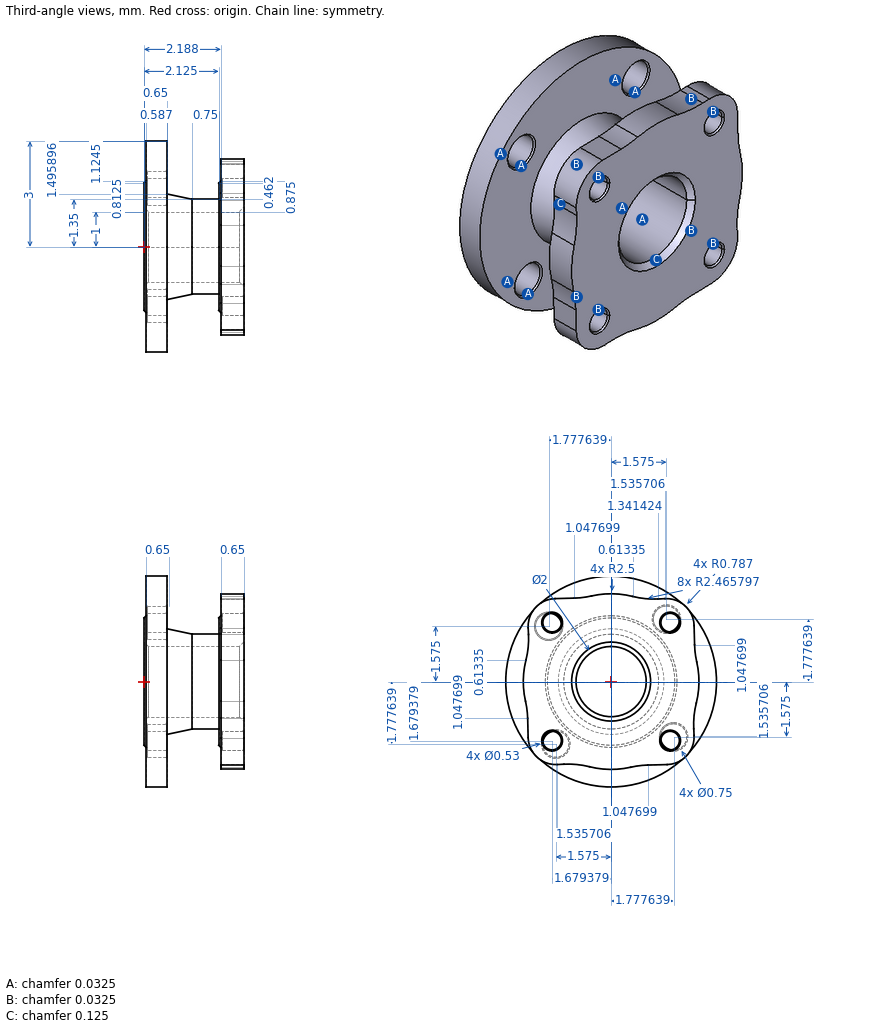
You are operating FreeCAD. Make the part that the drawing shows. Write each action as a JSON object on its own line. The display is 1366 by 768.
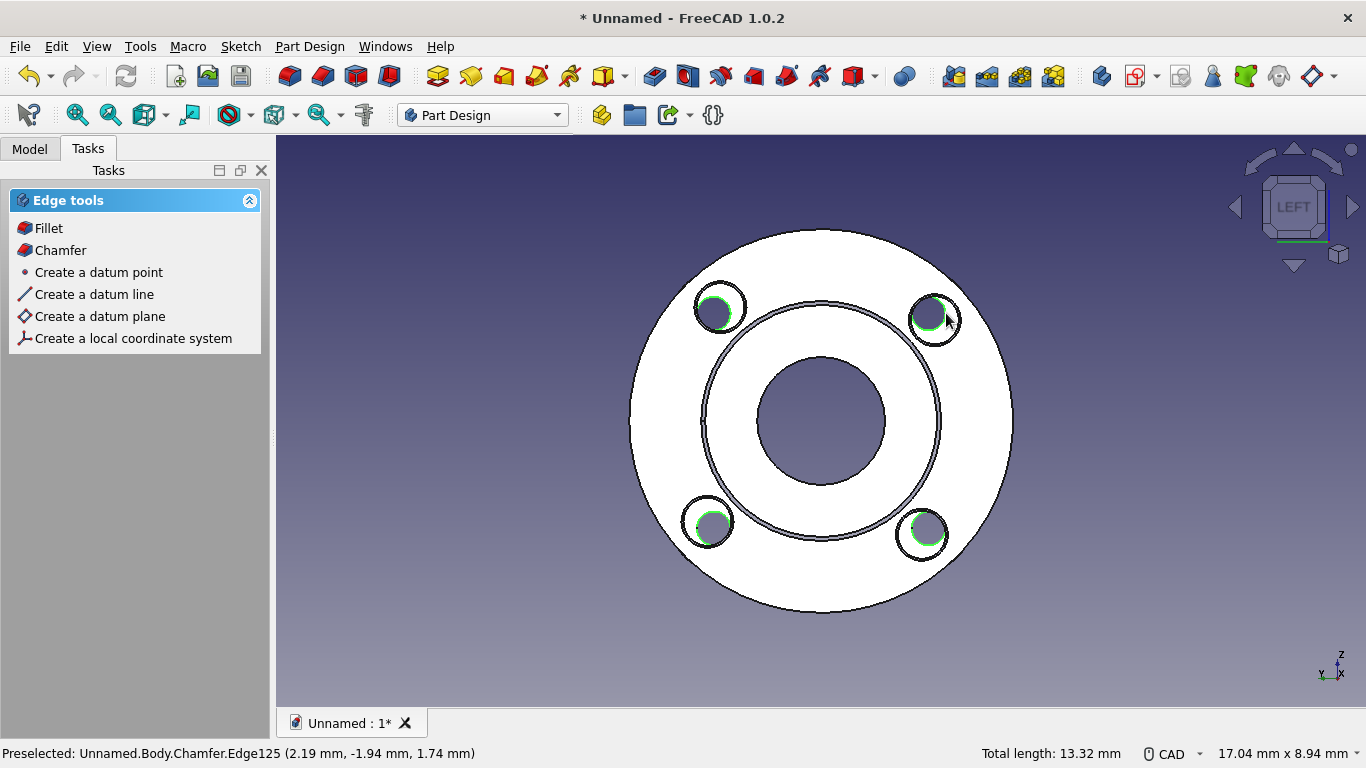
{"action": "left_click", "coordinate": [323, 76]}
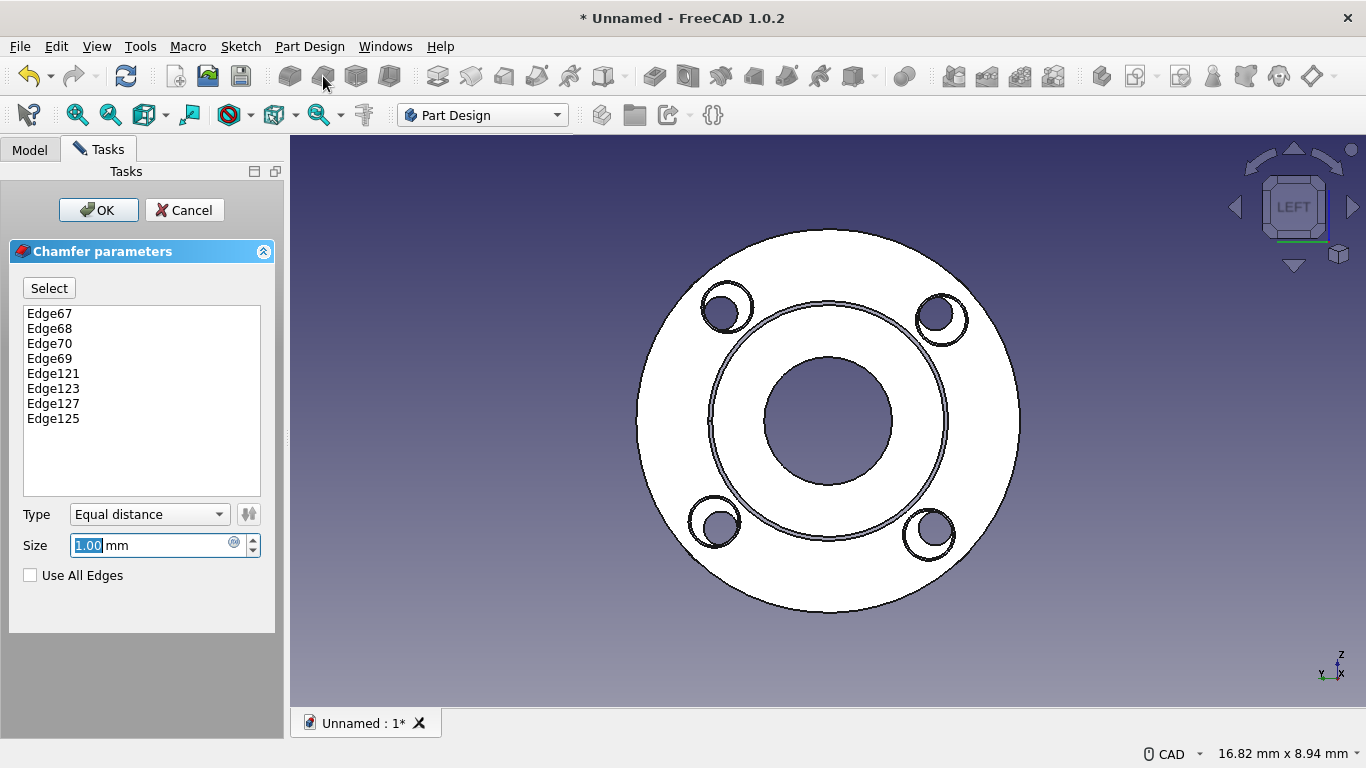
{"action": "type", "text": "0.0325"}
{"action": "key", "text": "Tab"}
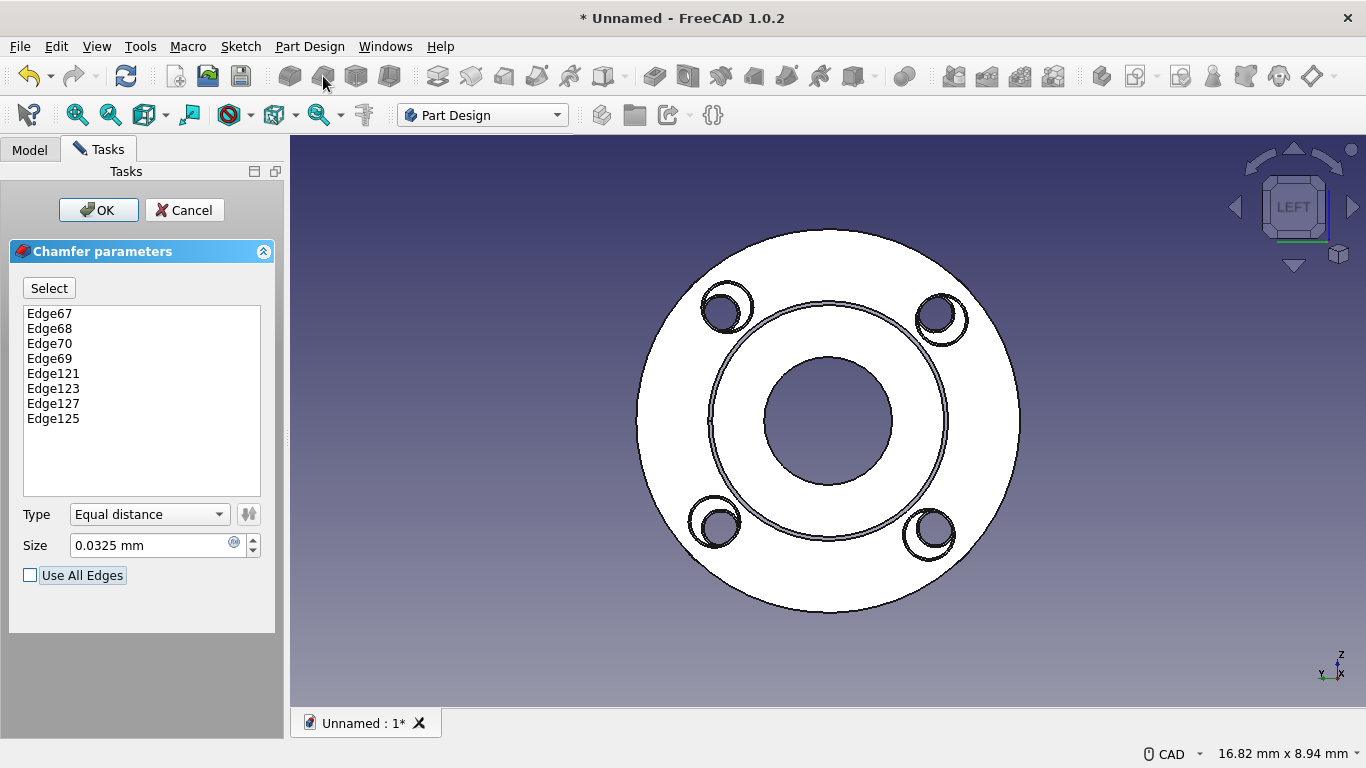
{"action": "left_click", "coordinate": [99, 210]}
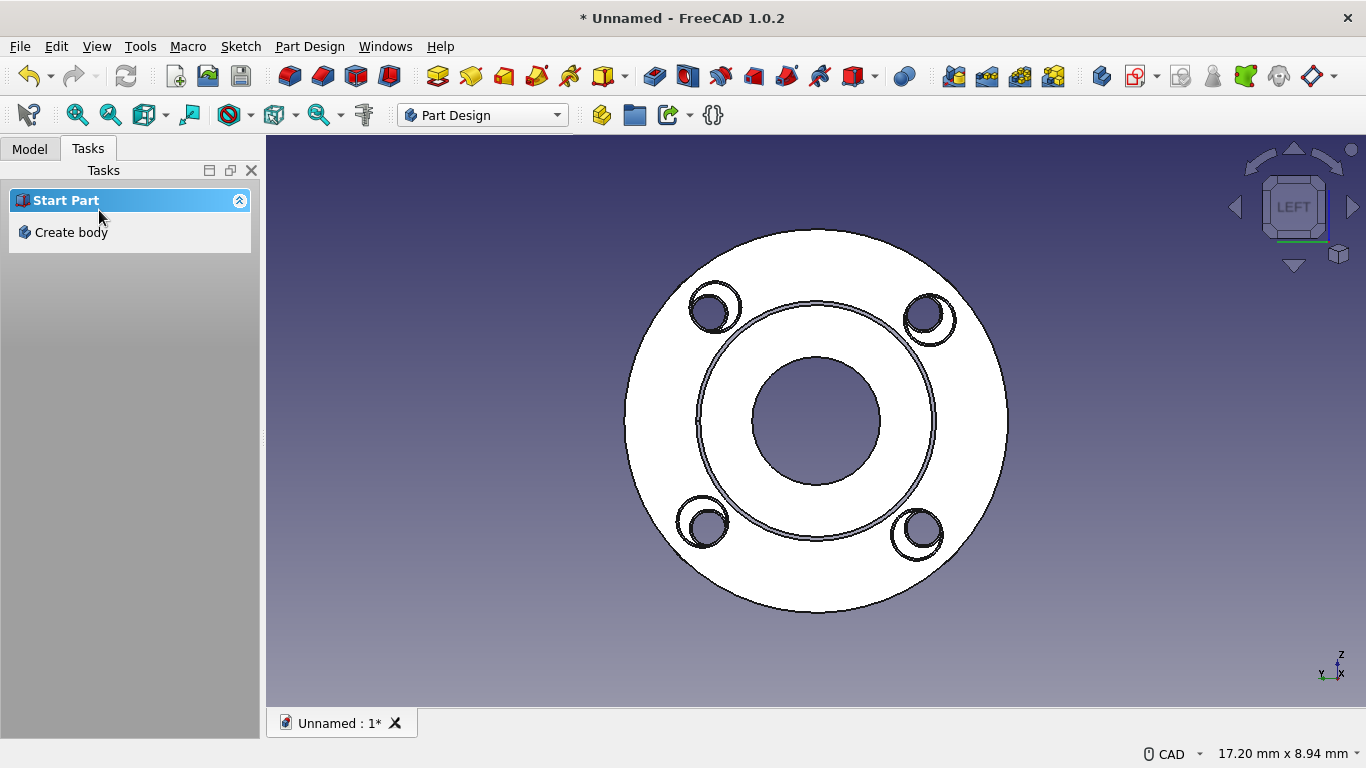
{"action": "left_click", "coordinate": [880, 420]}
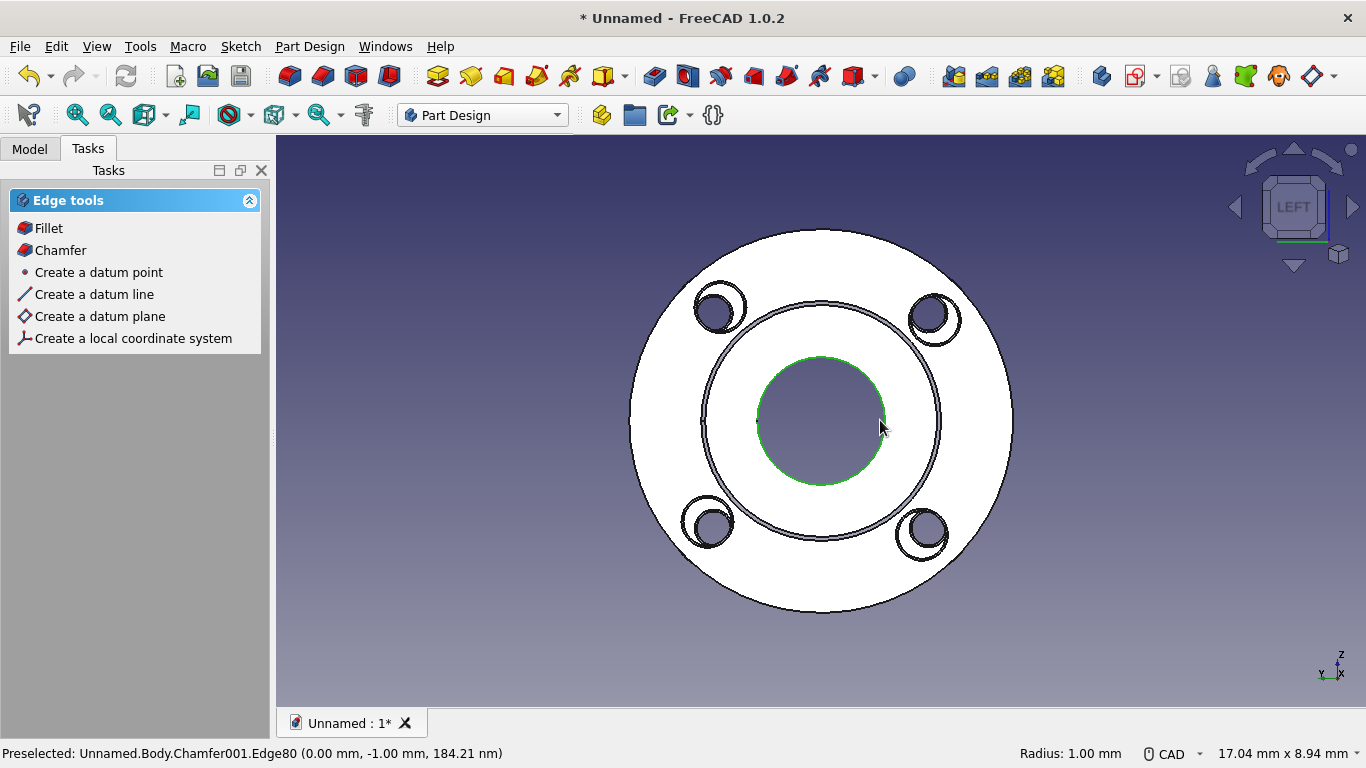
{"action": "key", "text": "0"}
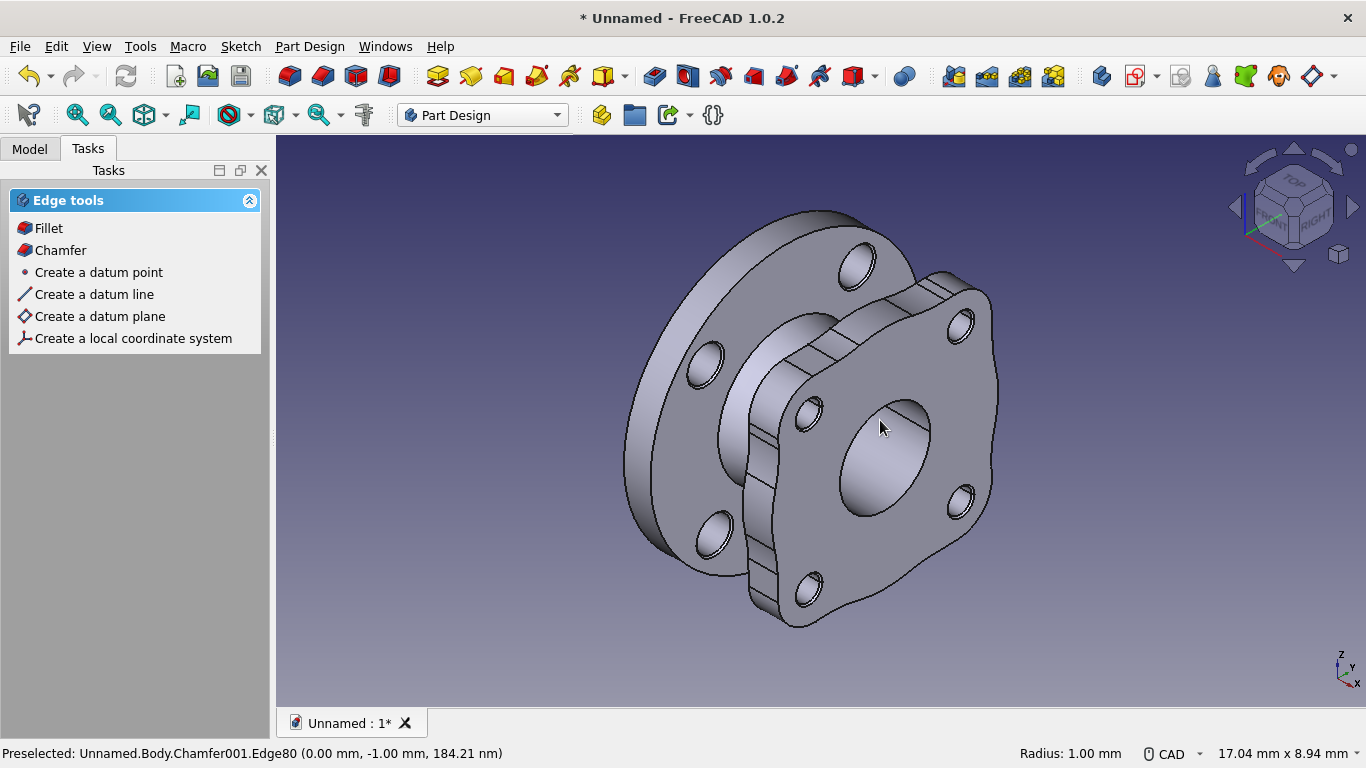
{"action": "left_click", "coordinate": [871, 416], "text": "ctrl"}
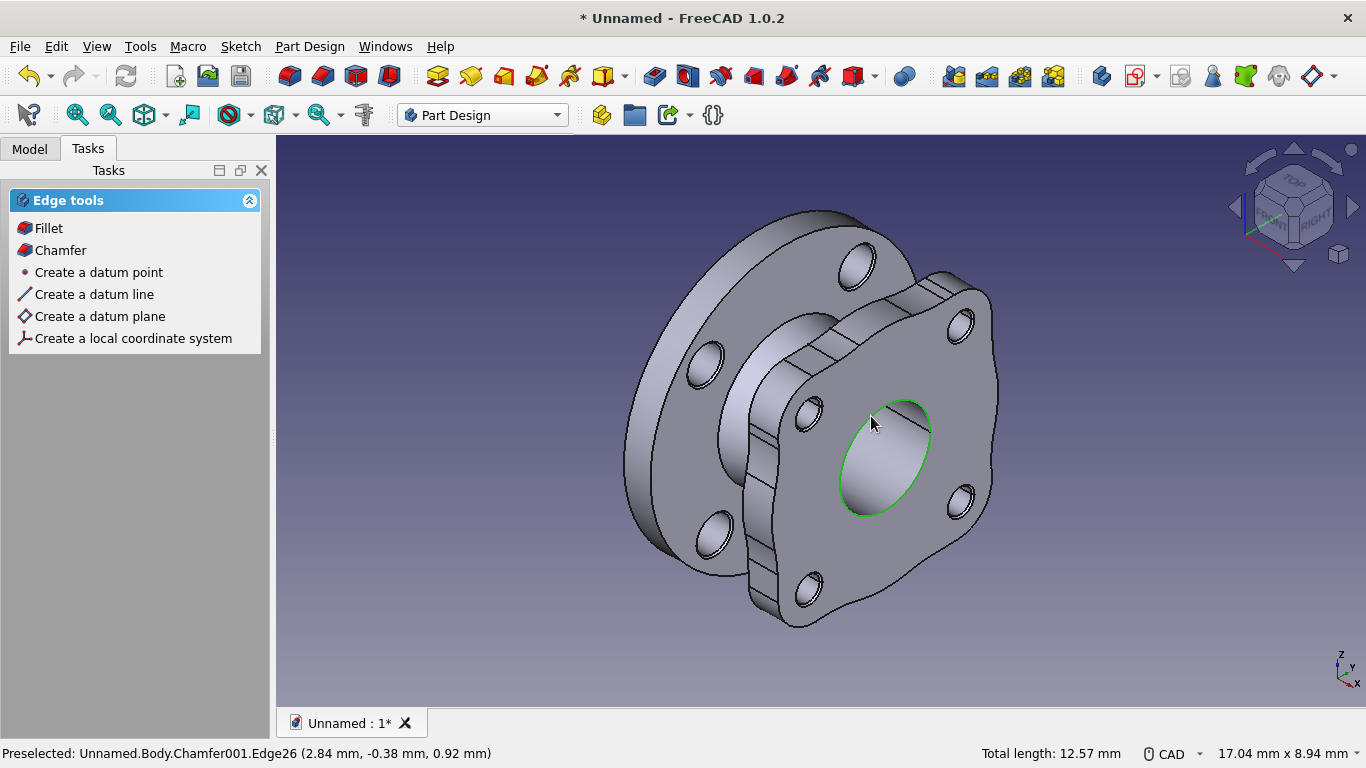
{"action": "left_click", "coordinate": [323, 76]}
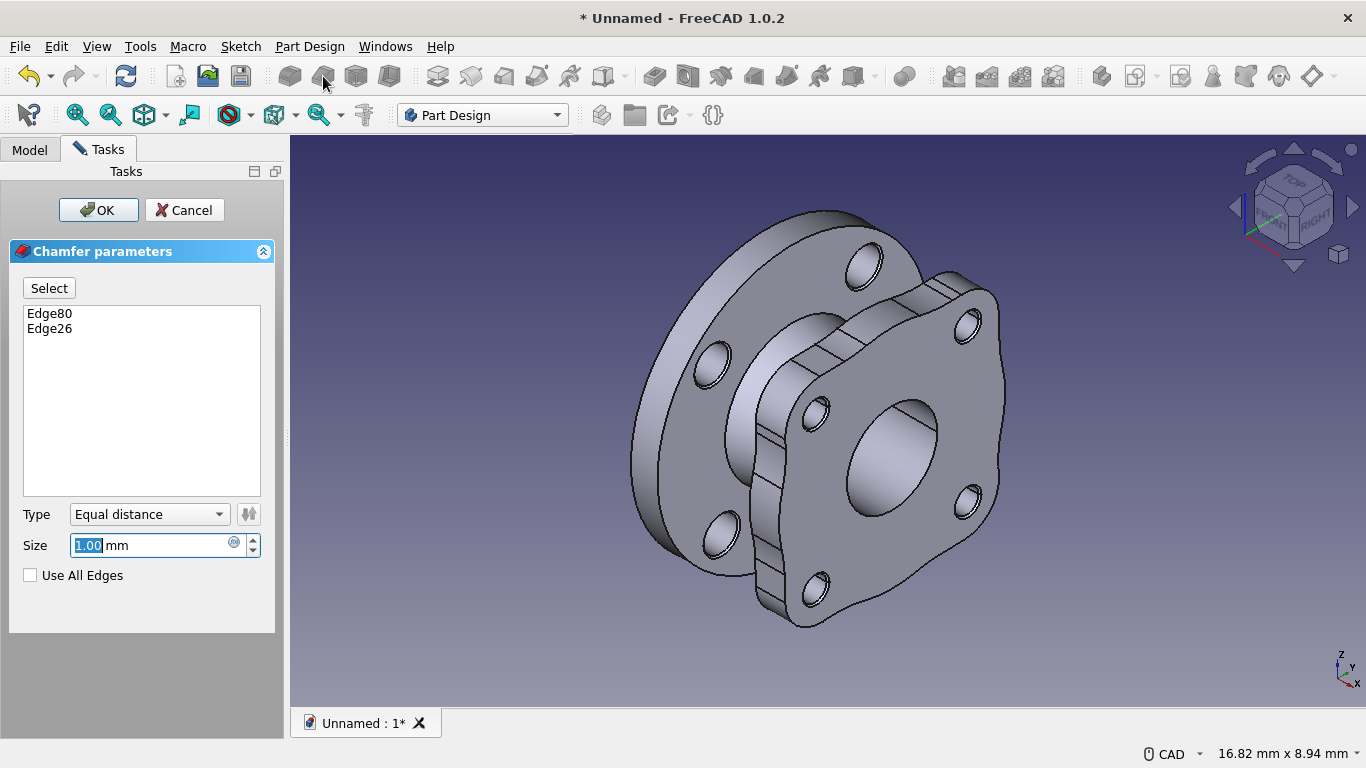
{"action": "type", "text": "0.125"}
{"action": "key", "text": "Tab"}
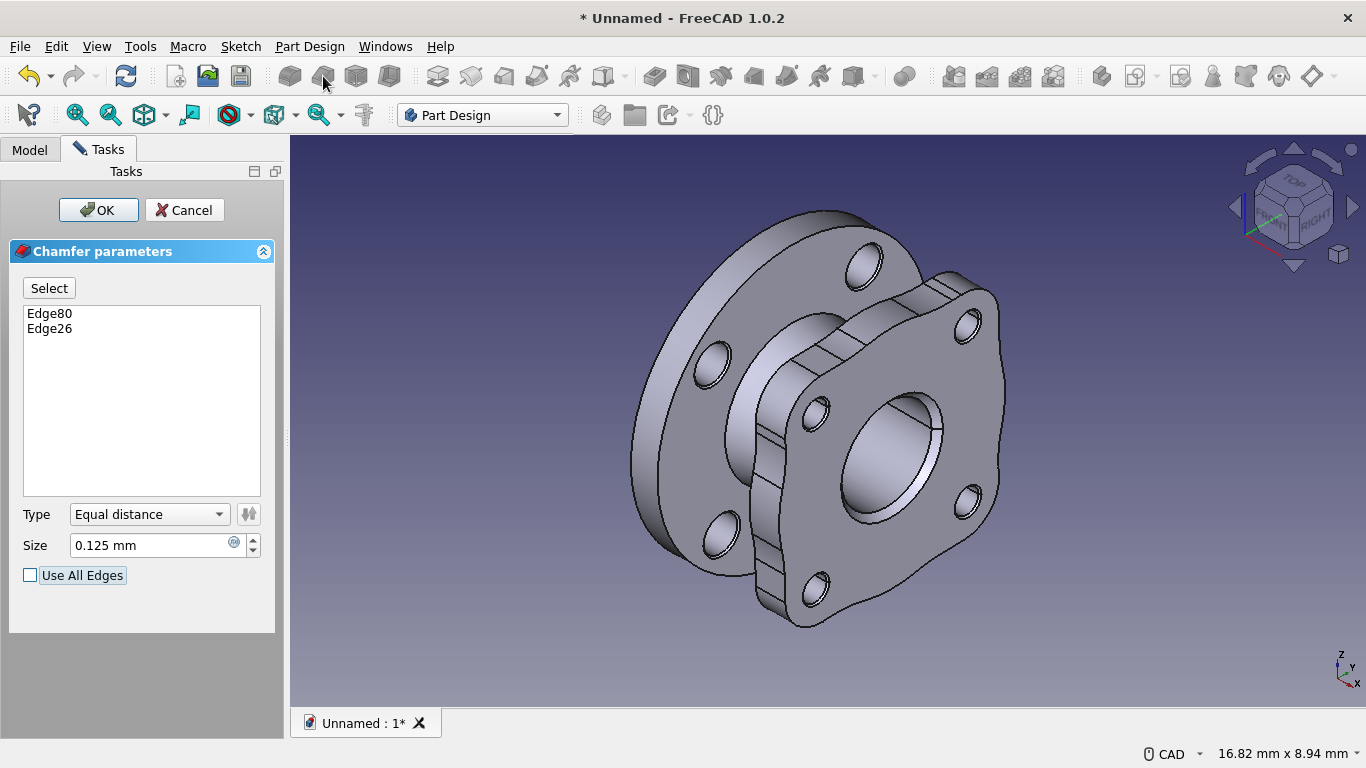
{"action": "left_click", "coordinate": [99, 210]}